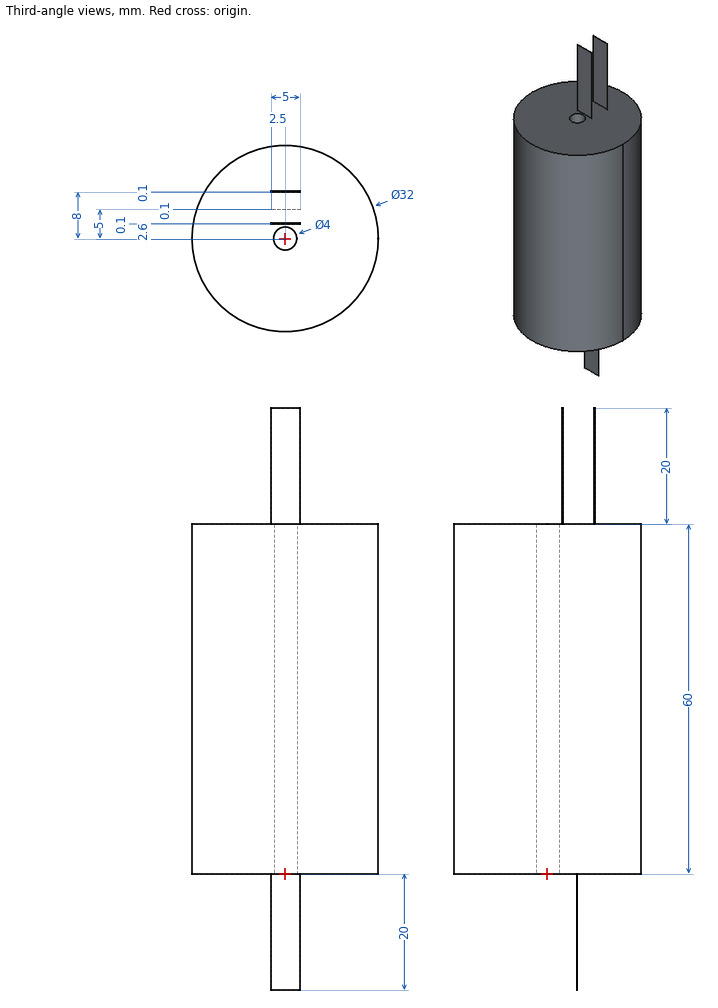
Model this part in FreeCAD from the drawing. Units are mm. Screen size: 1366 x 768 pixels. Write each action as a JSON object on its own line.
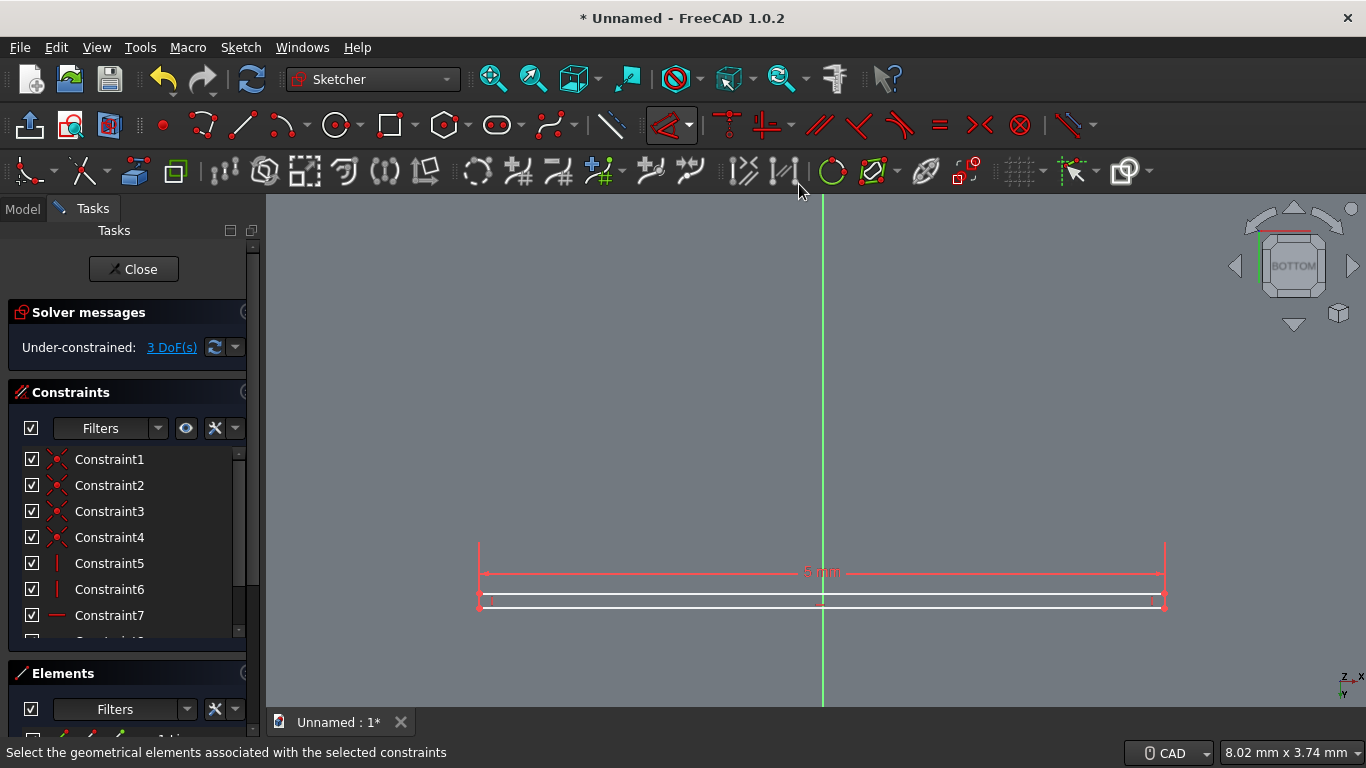
{"action": "left_click", "coordinate": [479, 594]}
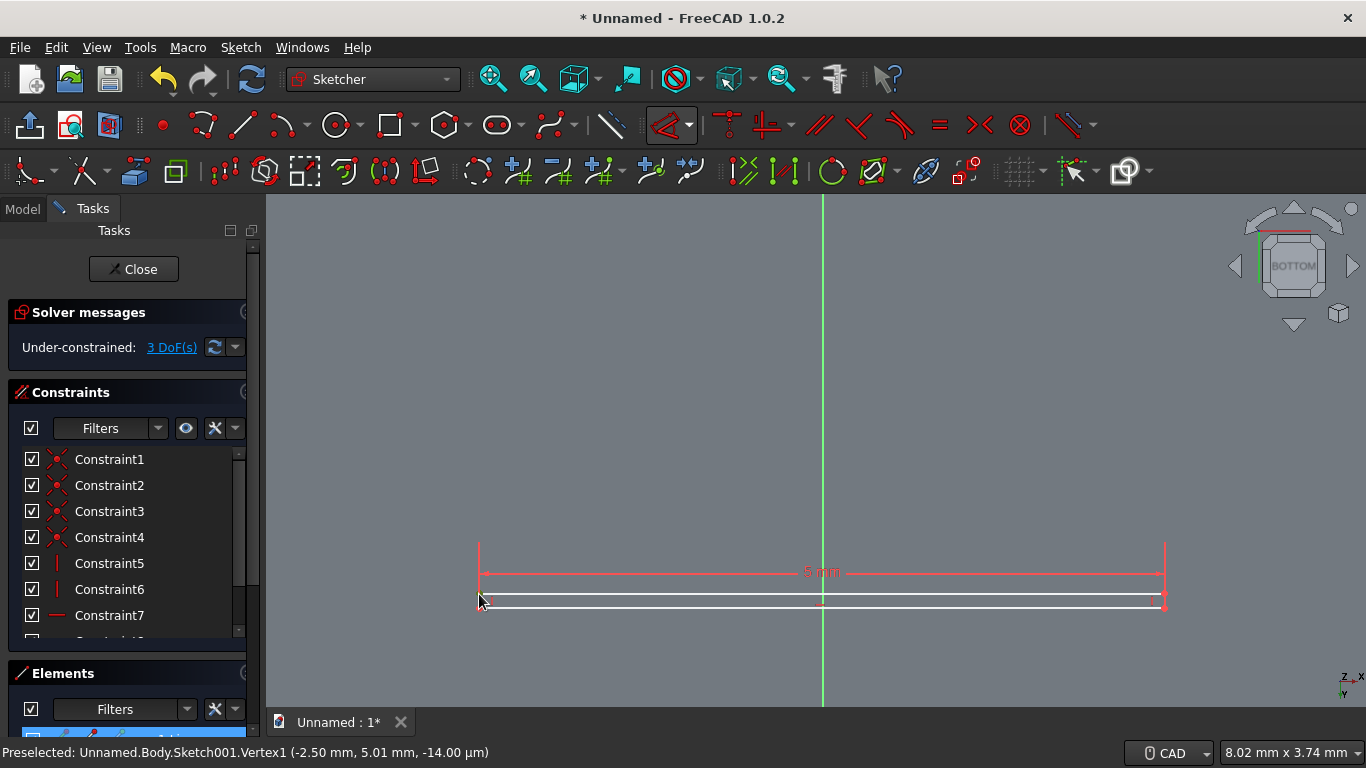
{"action": "left_click", "coordinate": [692, 126]}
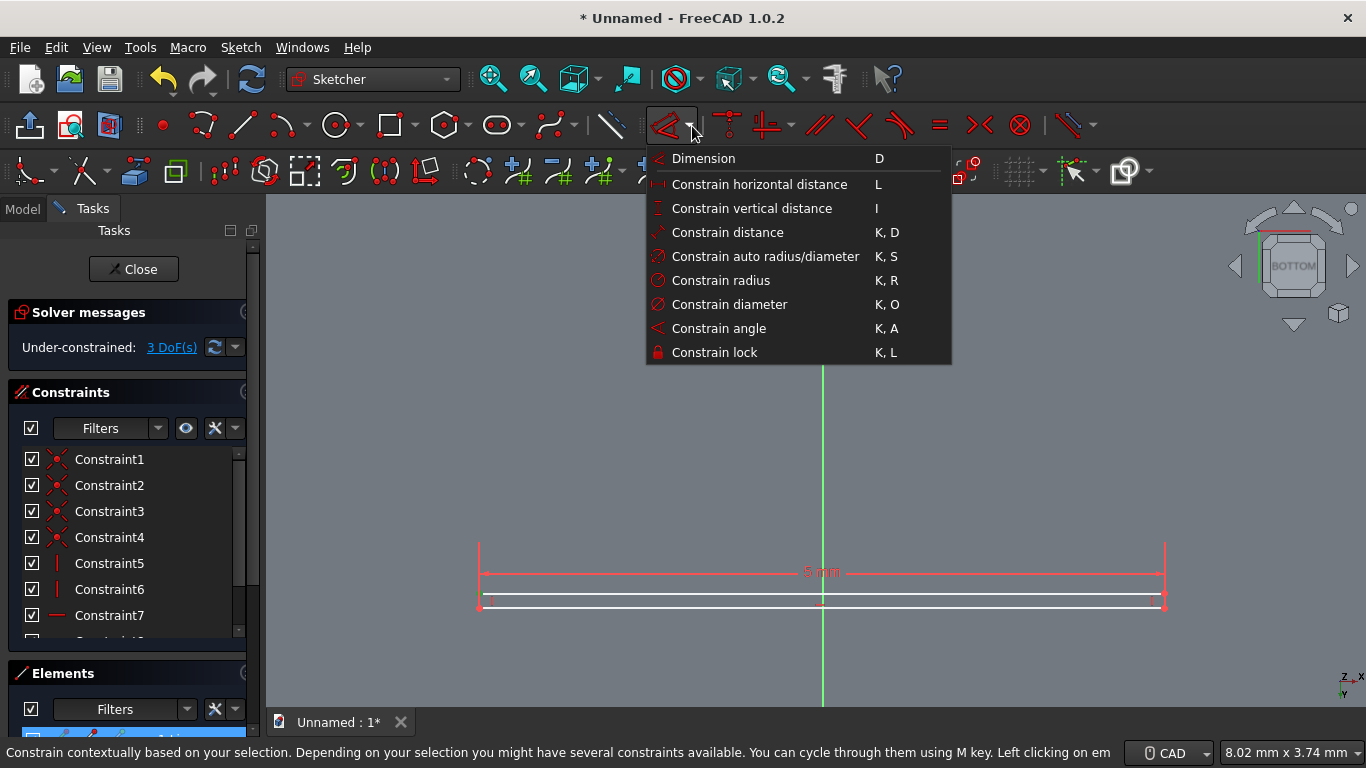
{"action": "left_click", "coordinate": [799, 208]}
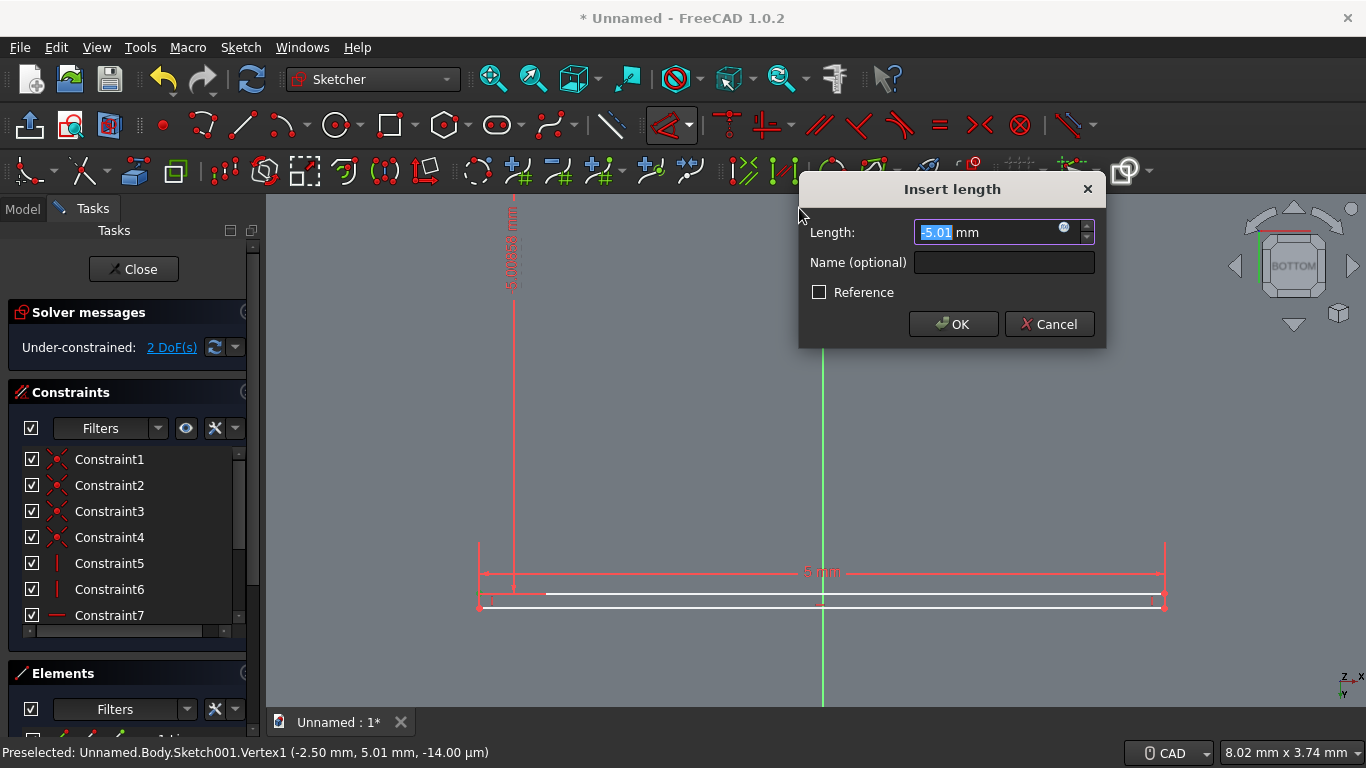
{"action": "type", "text": "-5"}
{"action": "key", "text": "Return"}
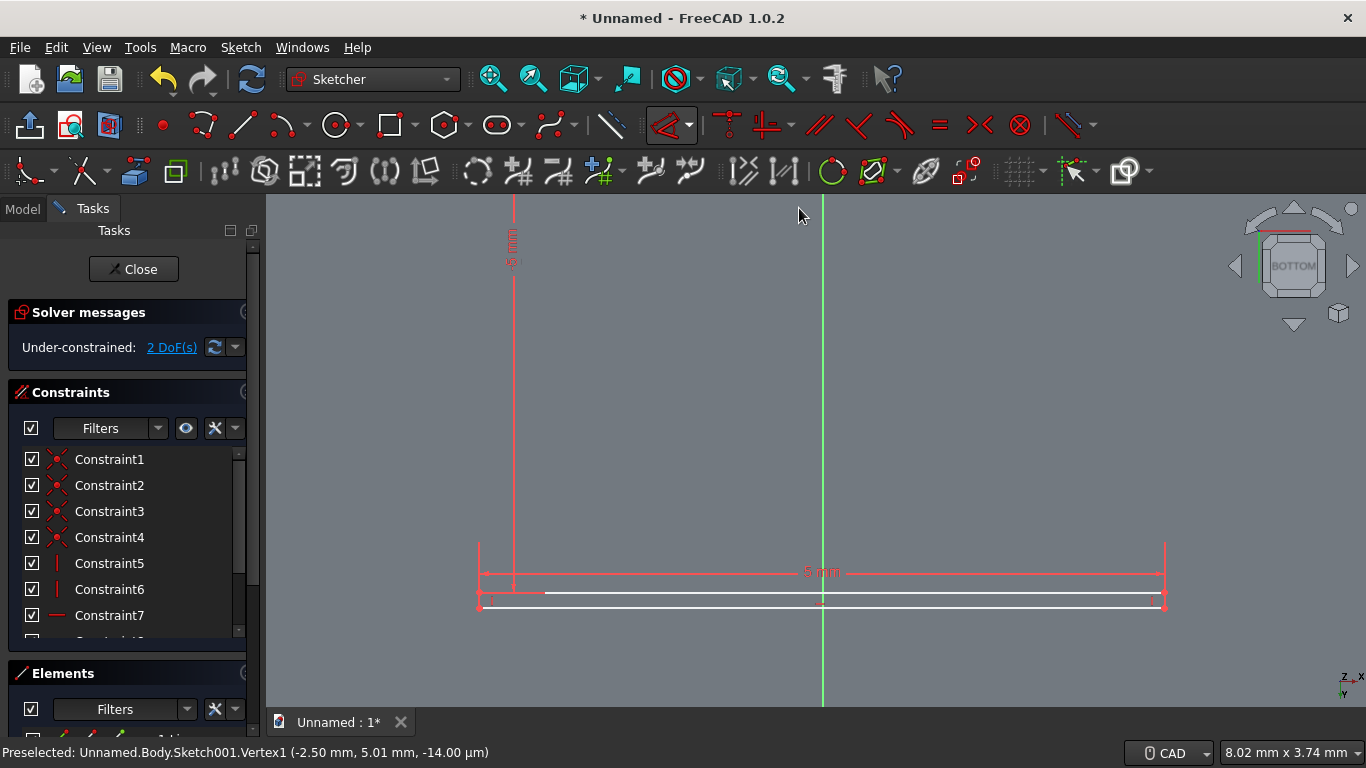
{"action": "scroll", "coordinate": [479, 600], "scroll_direction": "up", "scroll_amount": 6}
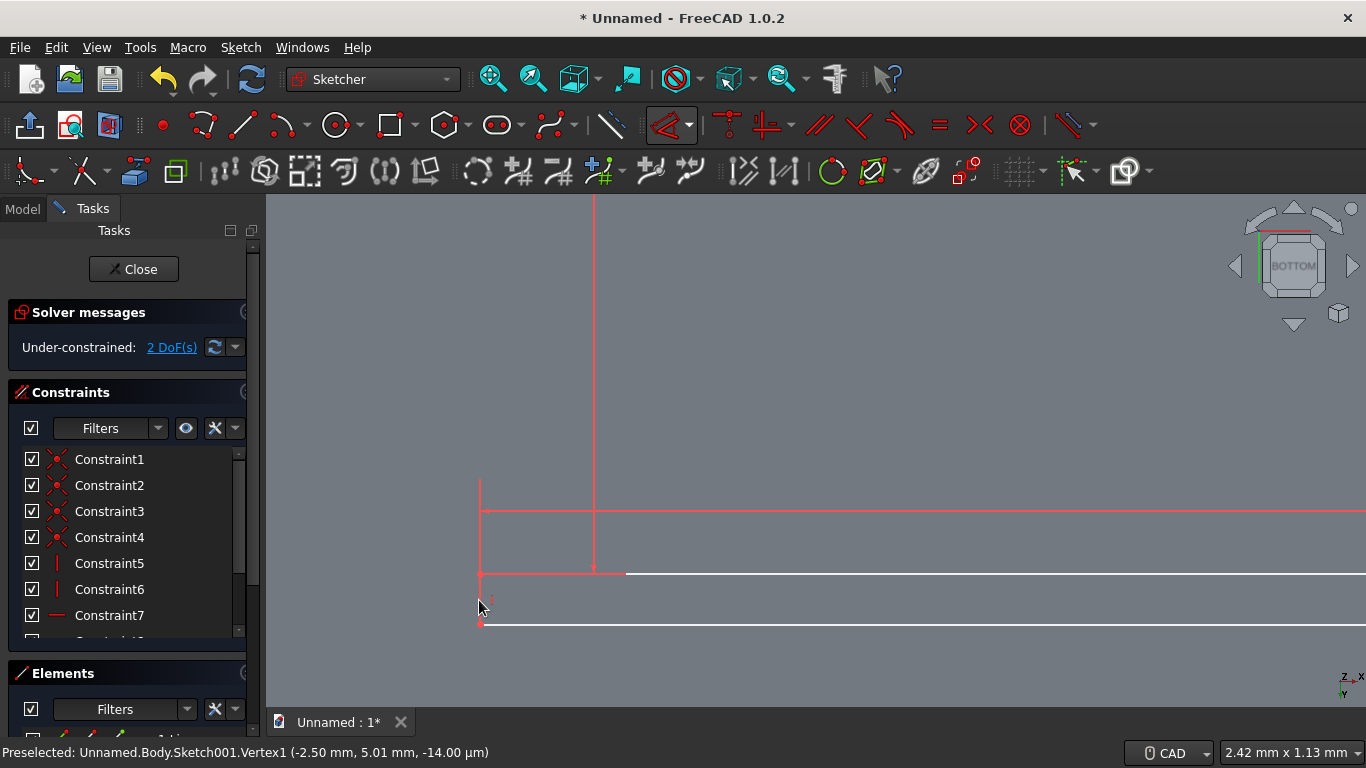
{"action": "left_click", "coordinate": [480, 599]}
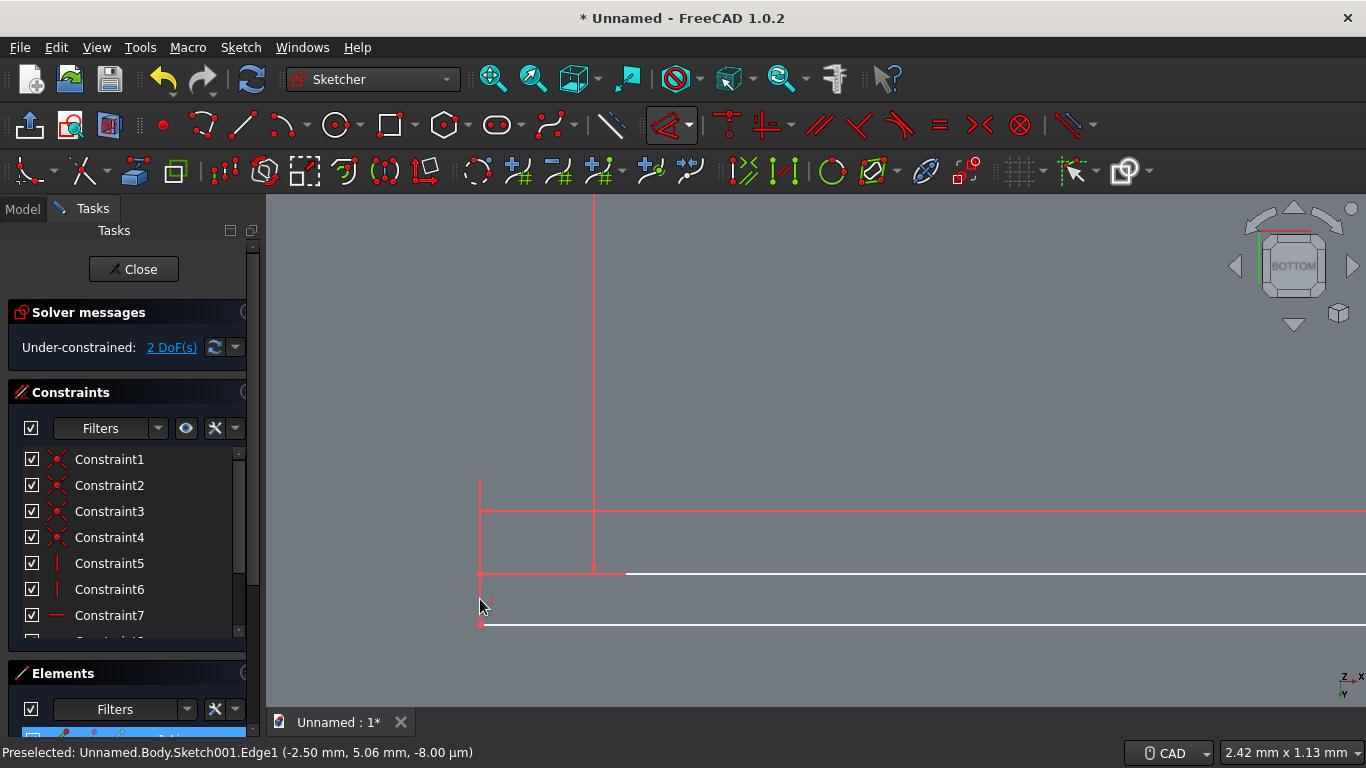
{"action": "left_click", "coordinate": [692, 126]}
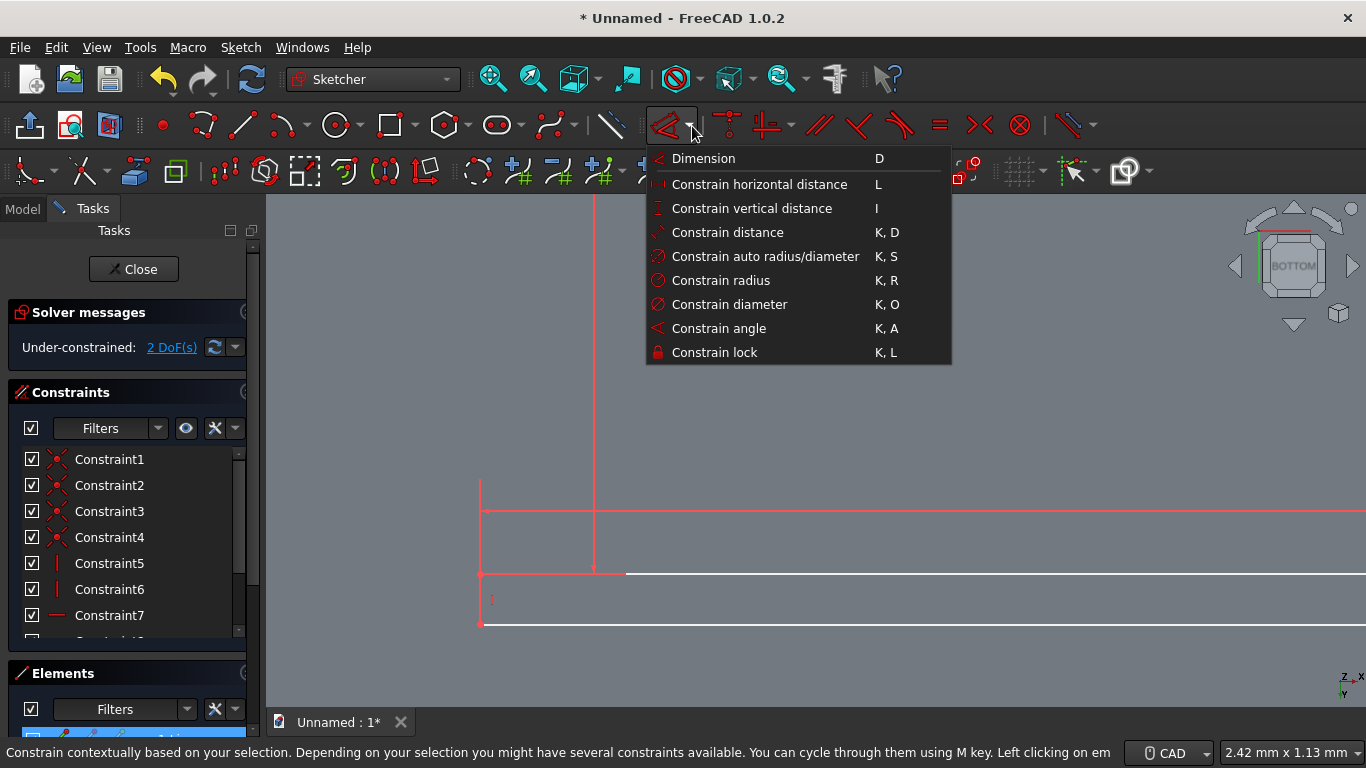
{"action": "left_click", "coordinate": [799, 208]}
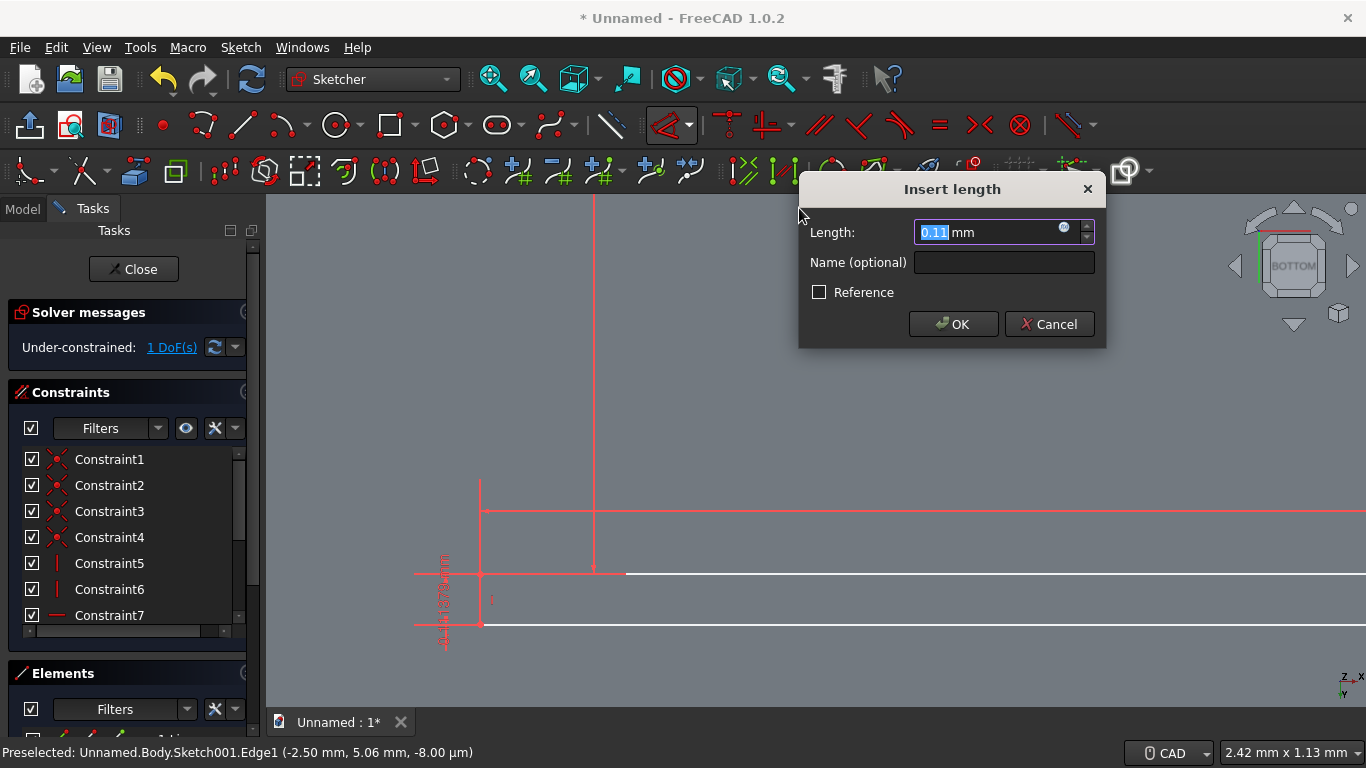
{"action": "type", "text": "0.1"}
{"action": "key", "text": "Return"}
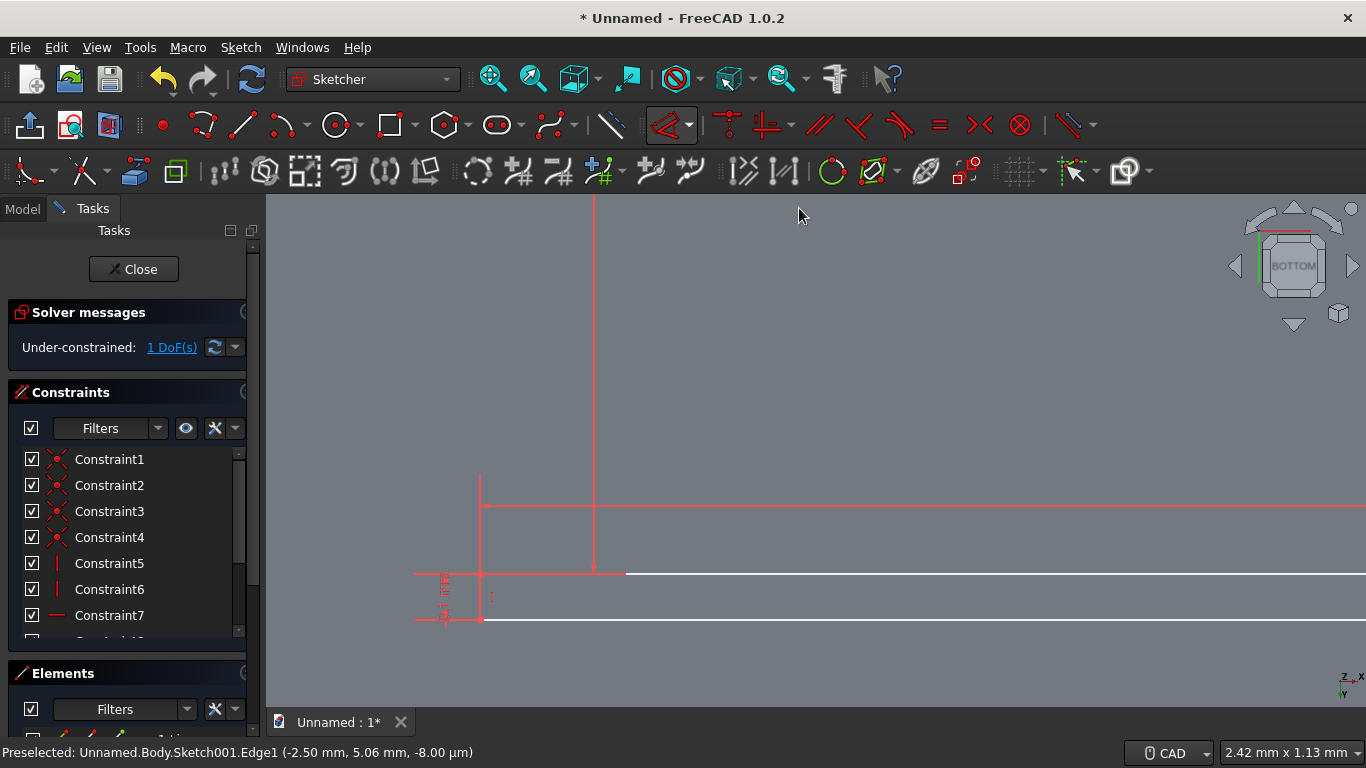
{"action": "scroll", "coordinate": [611, 606], "scroll_direction": "down", "scroll_amount": 10}